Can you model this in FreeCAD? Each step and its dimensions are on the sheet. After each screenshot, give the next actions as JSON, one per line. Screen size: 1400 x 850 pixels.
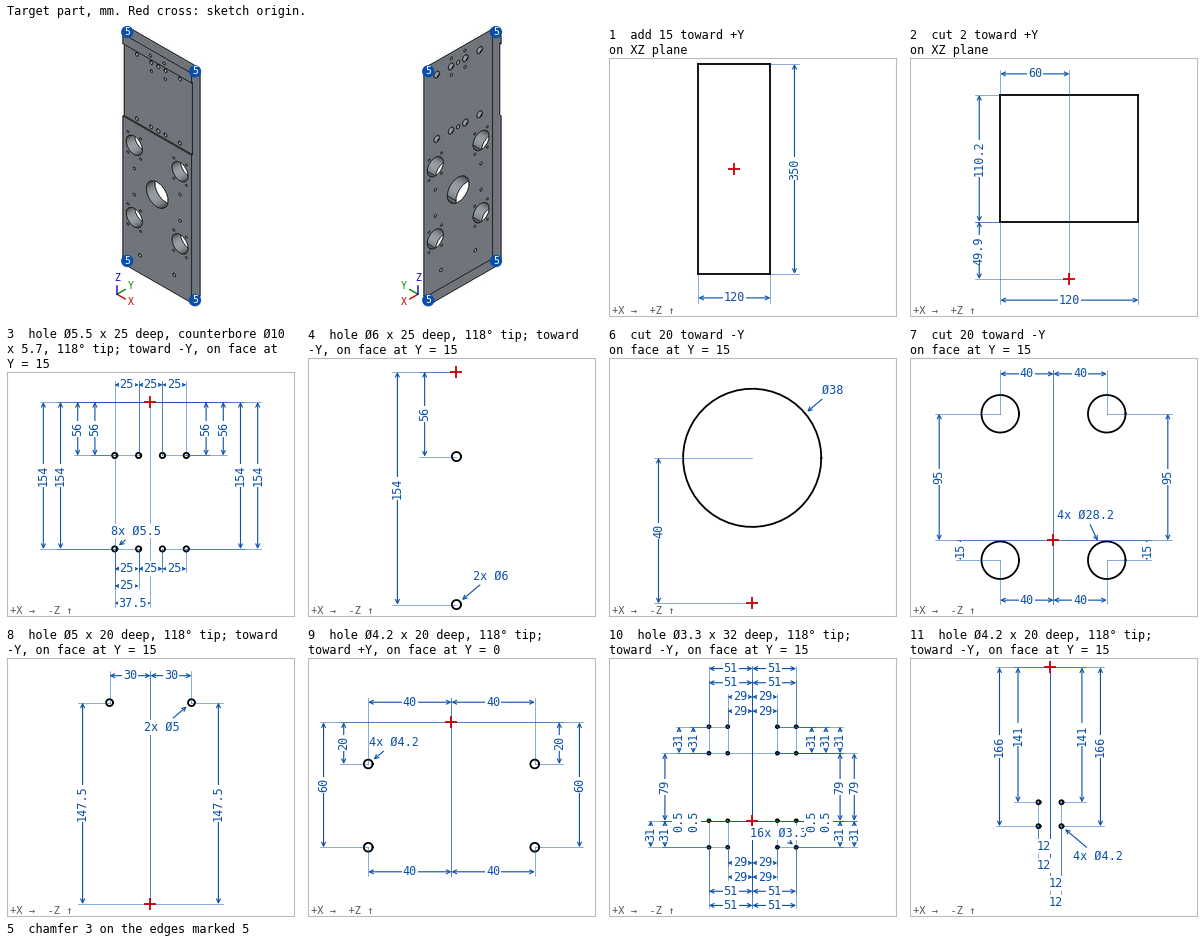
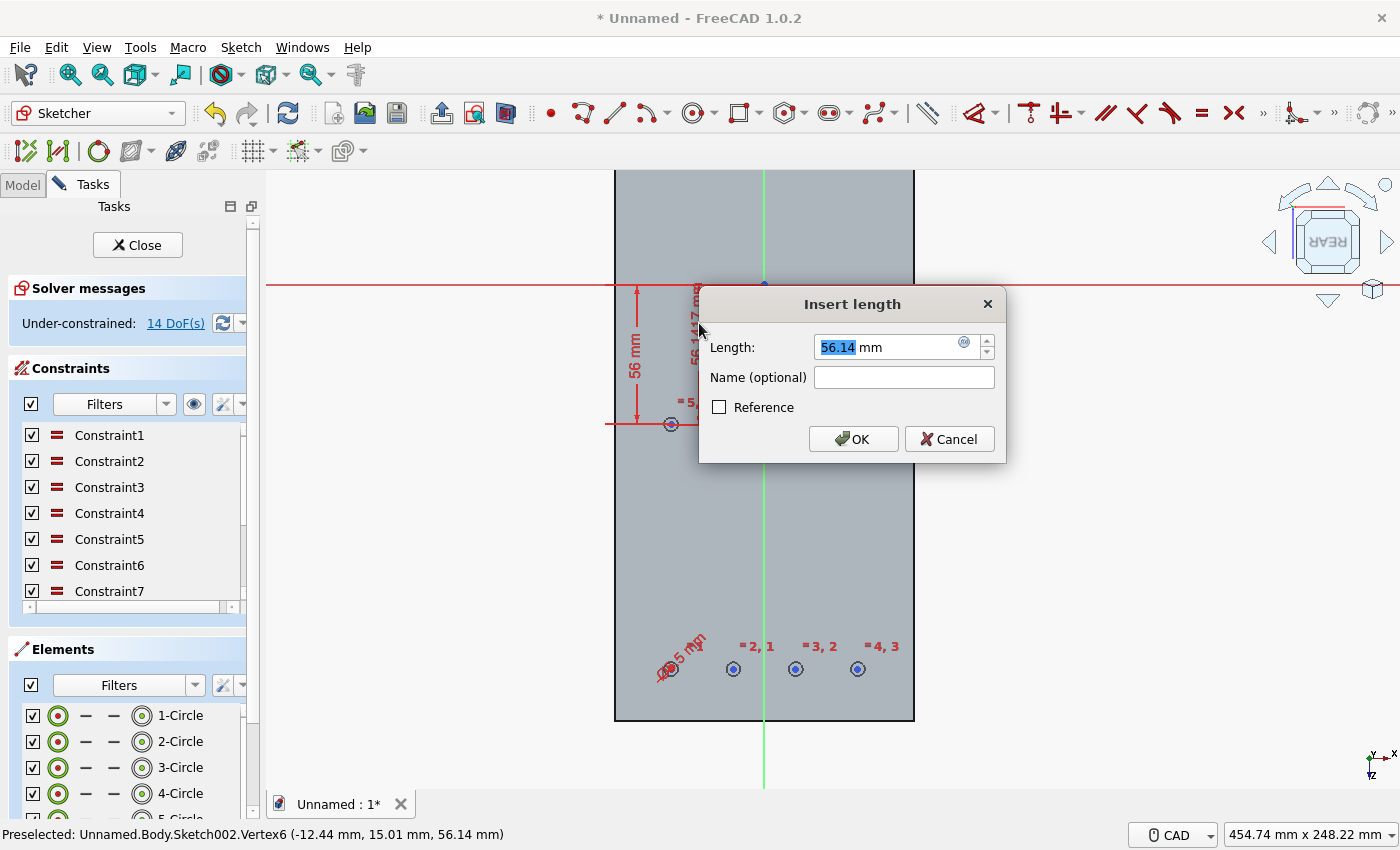
{"action": "type", "text": "56"}
{"action": "key", "text": "Return"}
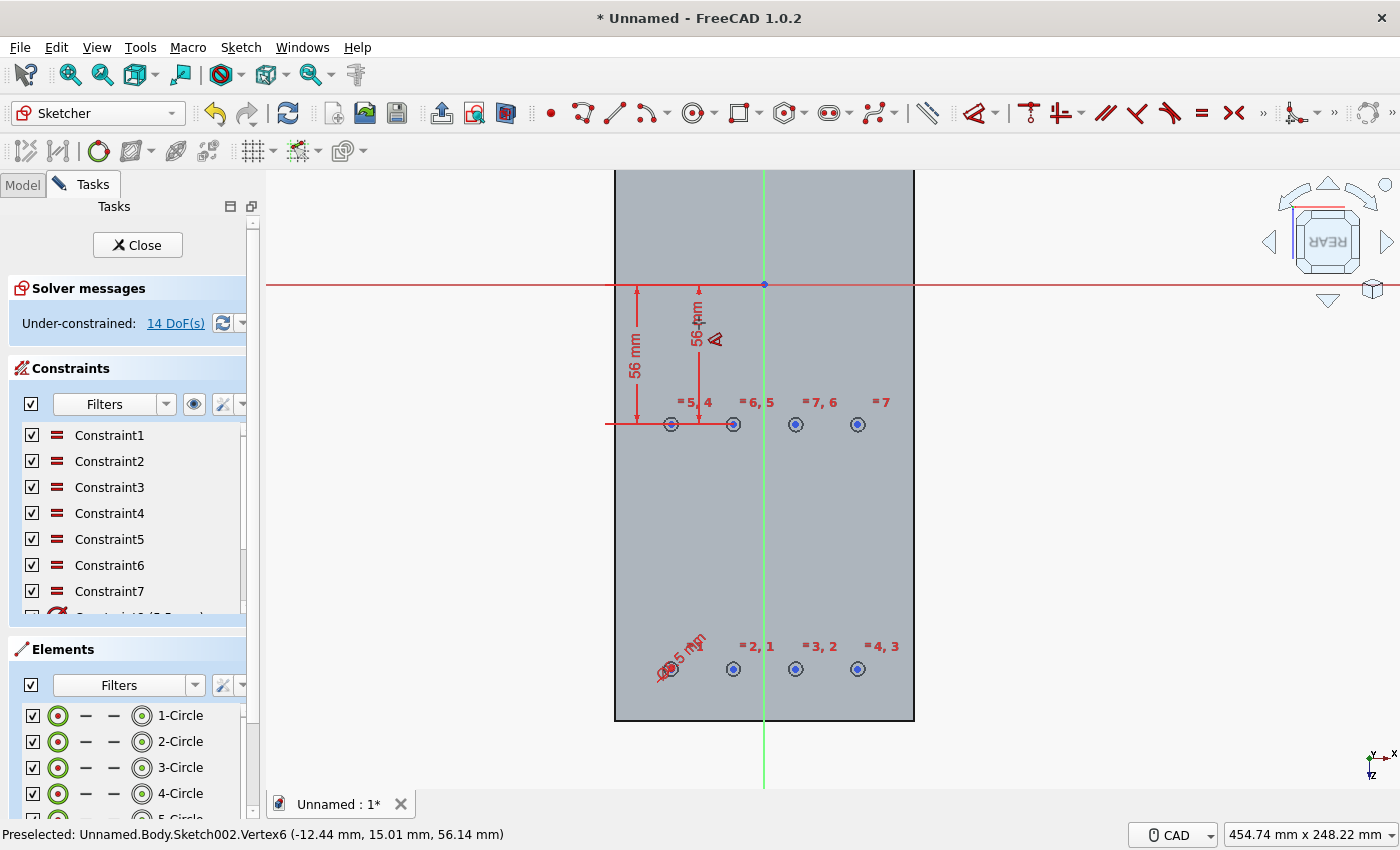
{"action": "left_click", "coordinate": [796, 425]}
{"action": "left_click", "coordinate": [830, 355]}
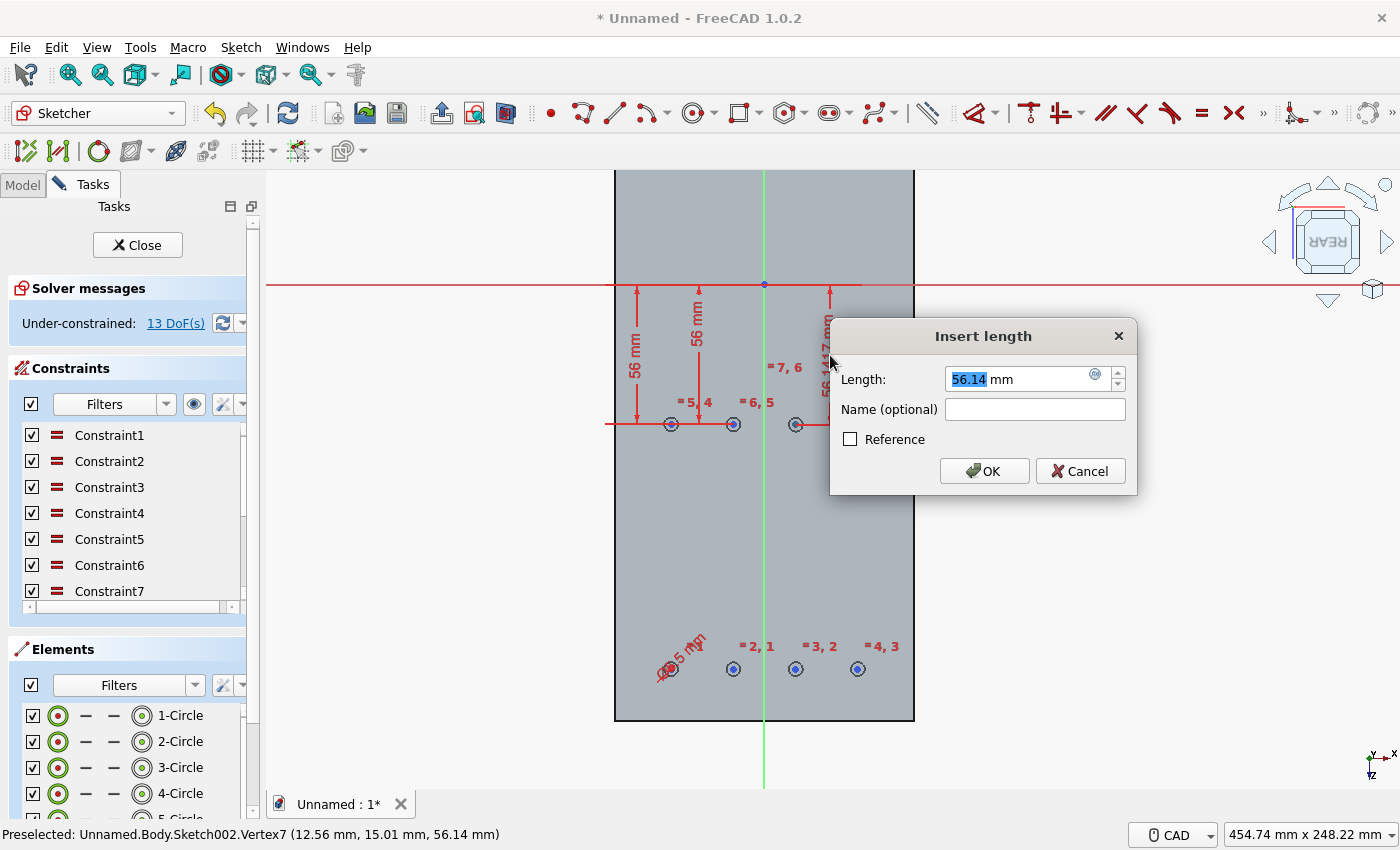
{"action": "type", "text": "56"}
{"action": "key", "text": "Return"}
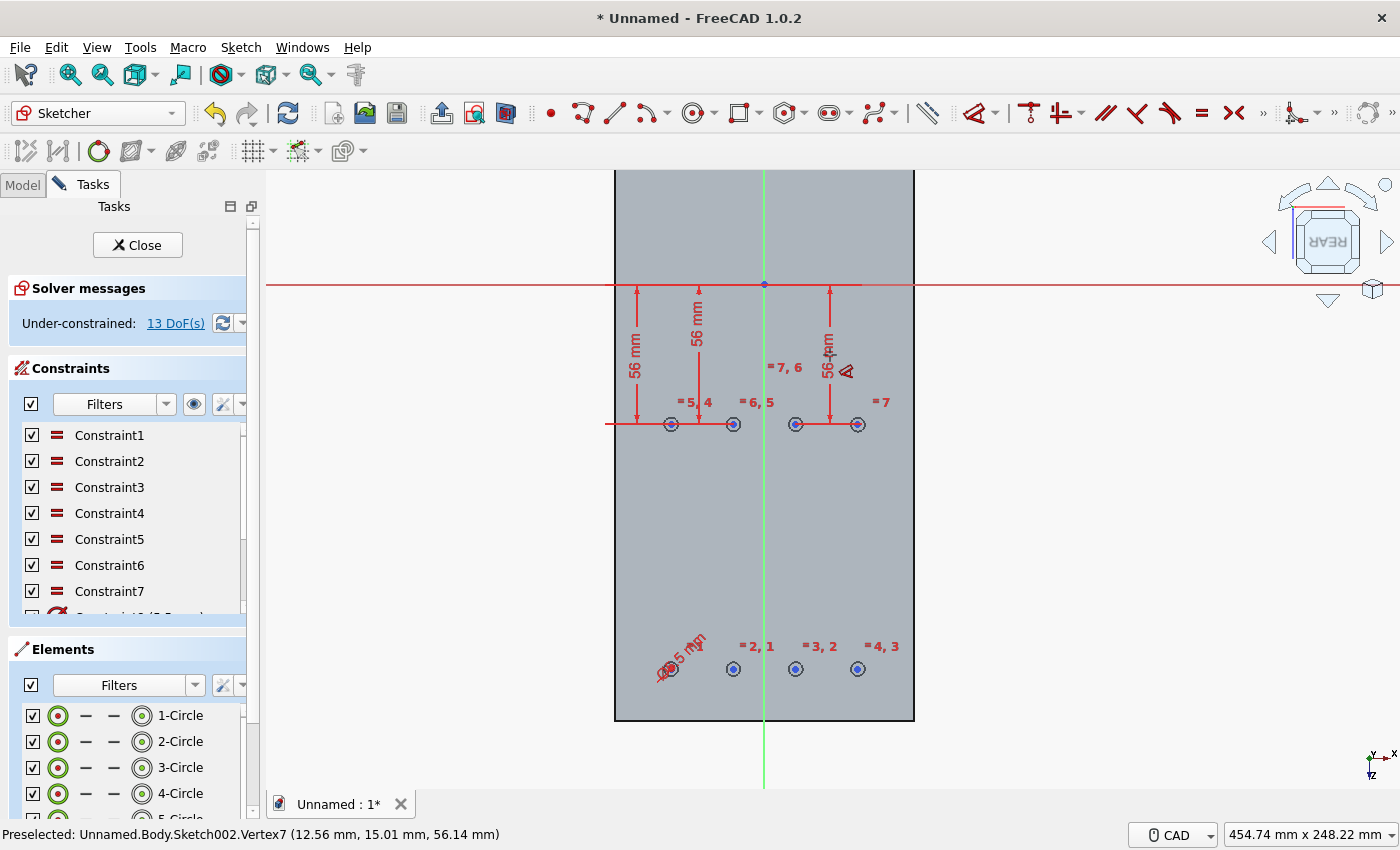
{"action": "left_click", "coordinate": [858, 425]}
{"action": "left_click", "coordinate": [892, 323]}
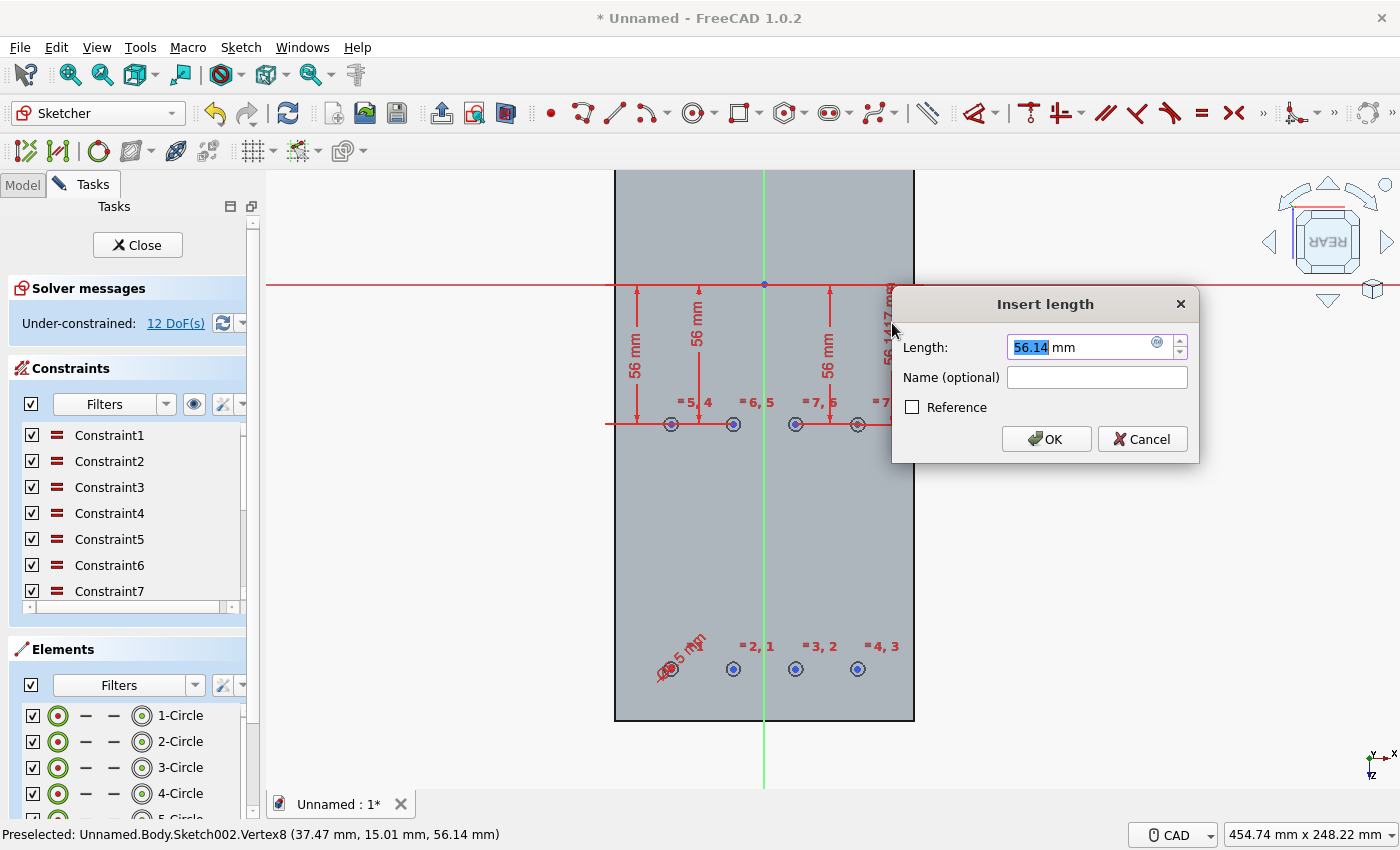
{"action": "type", "text": "56"}
{"action": "key", "text": "Return"}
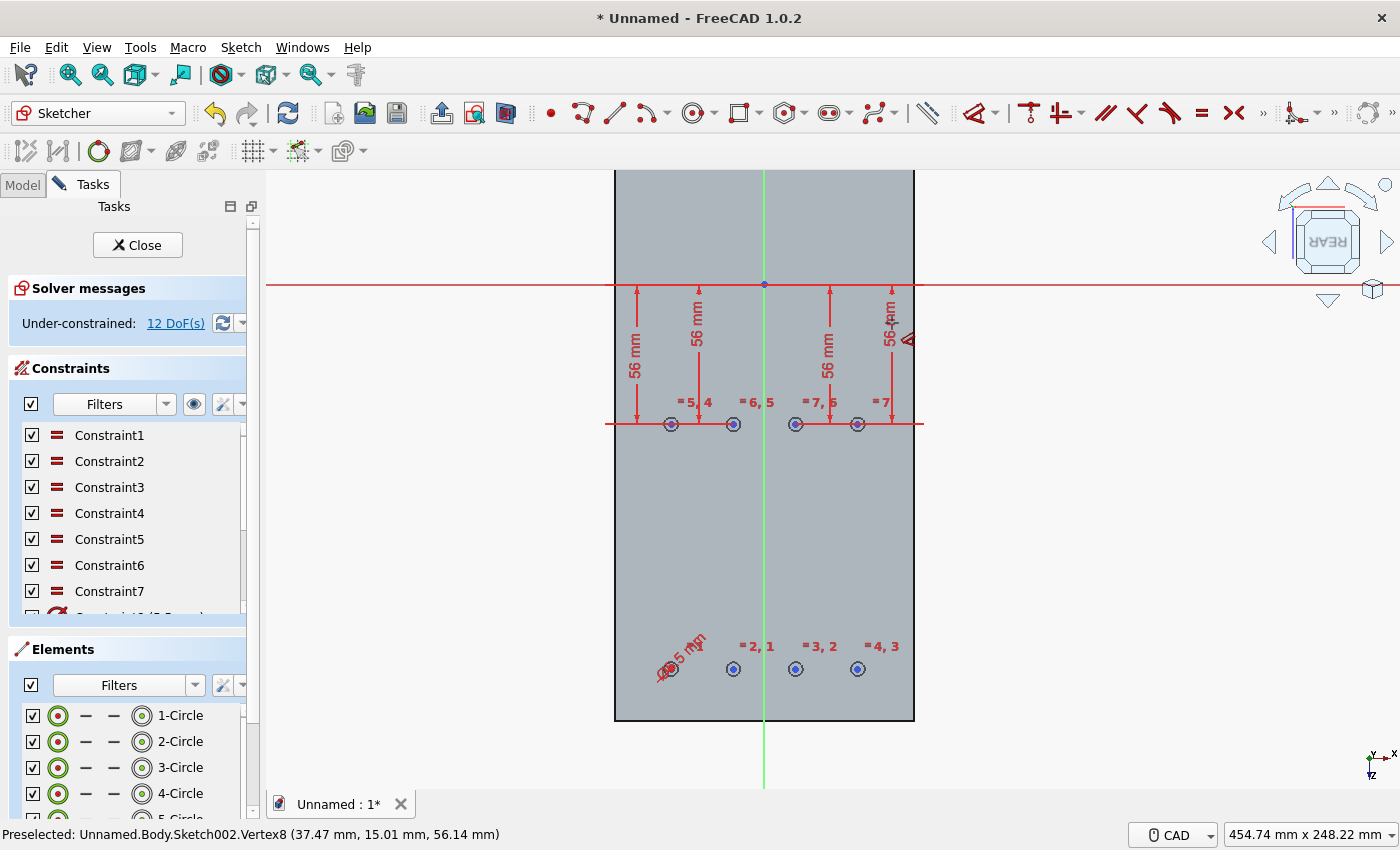
{"action": "left_click", "coordinate": [671, 669]}
{"action": "left_click", "coordinate": [637, 477]}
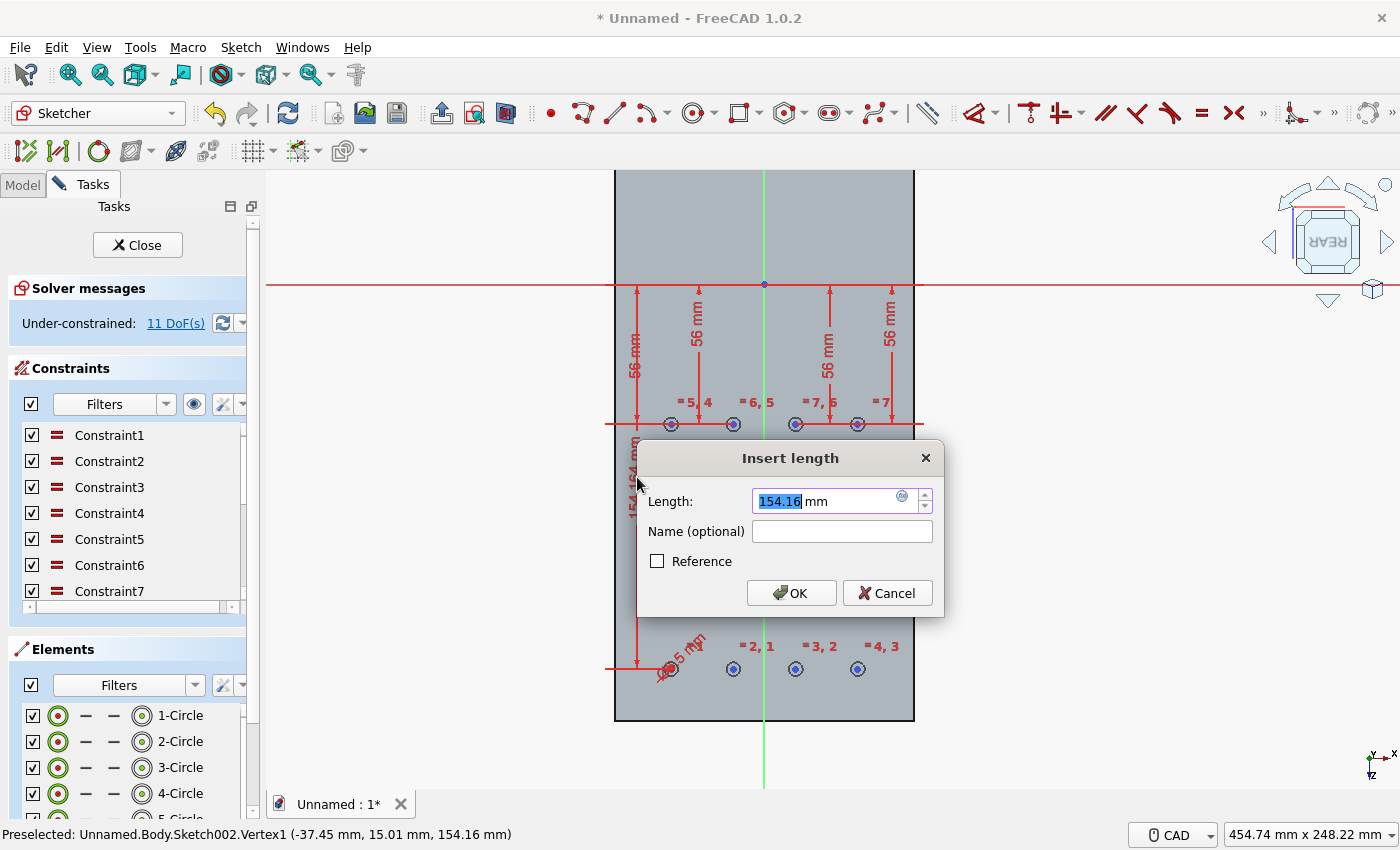
{"action": "type", "text": "154"}
{"action": "key", "text": "Return"}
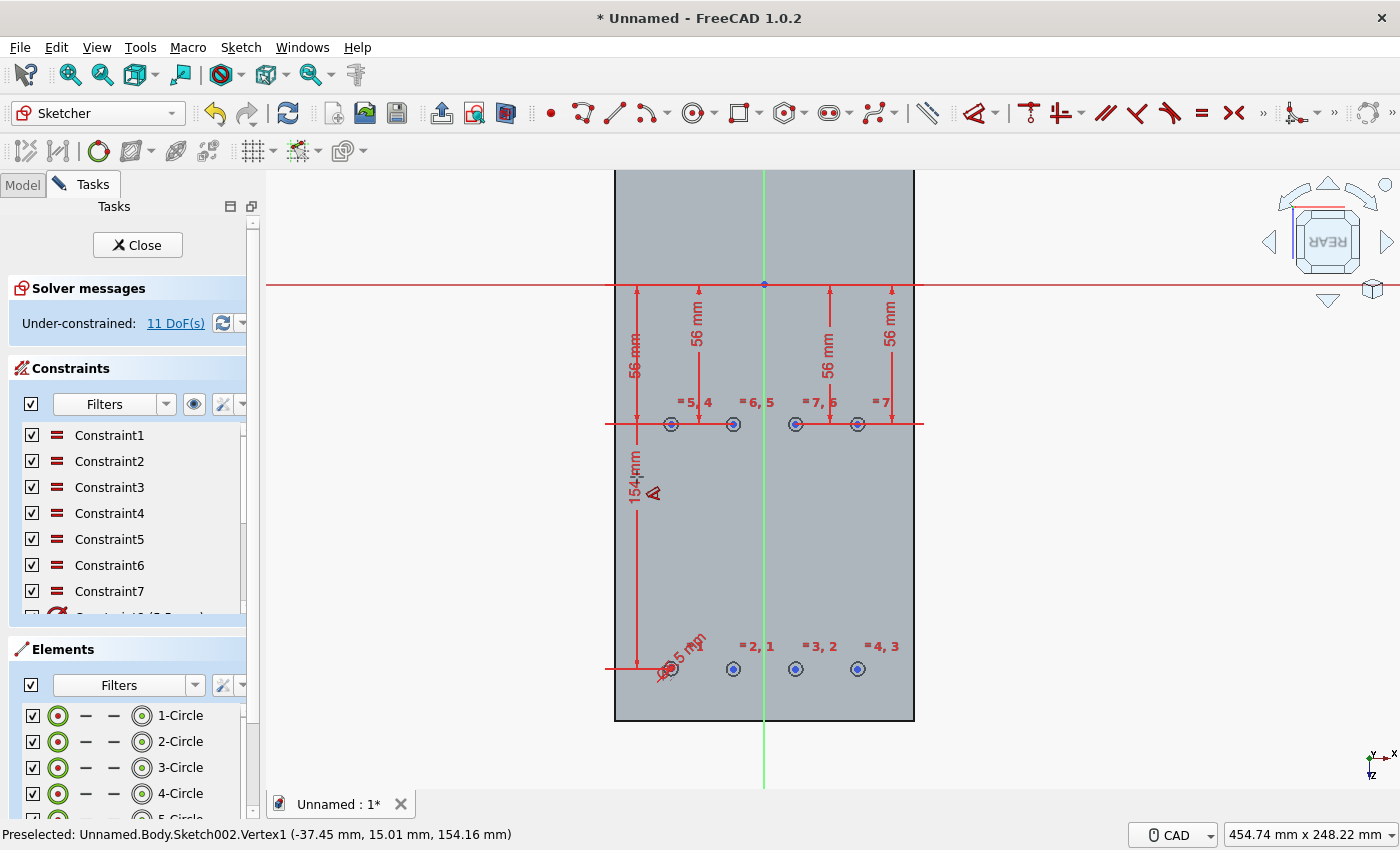
{"action": "left_click", "coordinate": [733, 669]}
{"action": "left_click", "coordinate": [699, 389]}